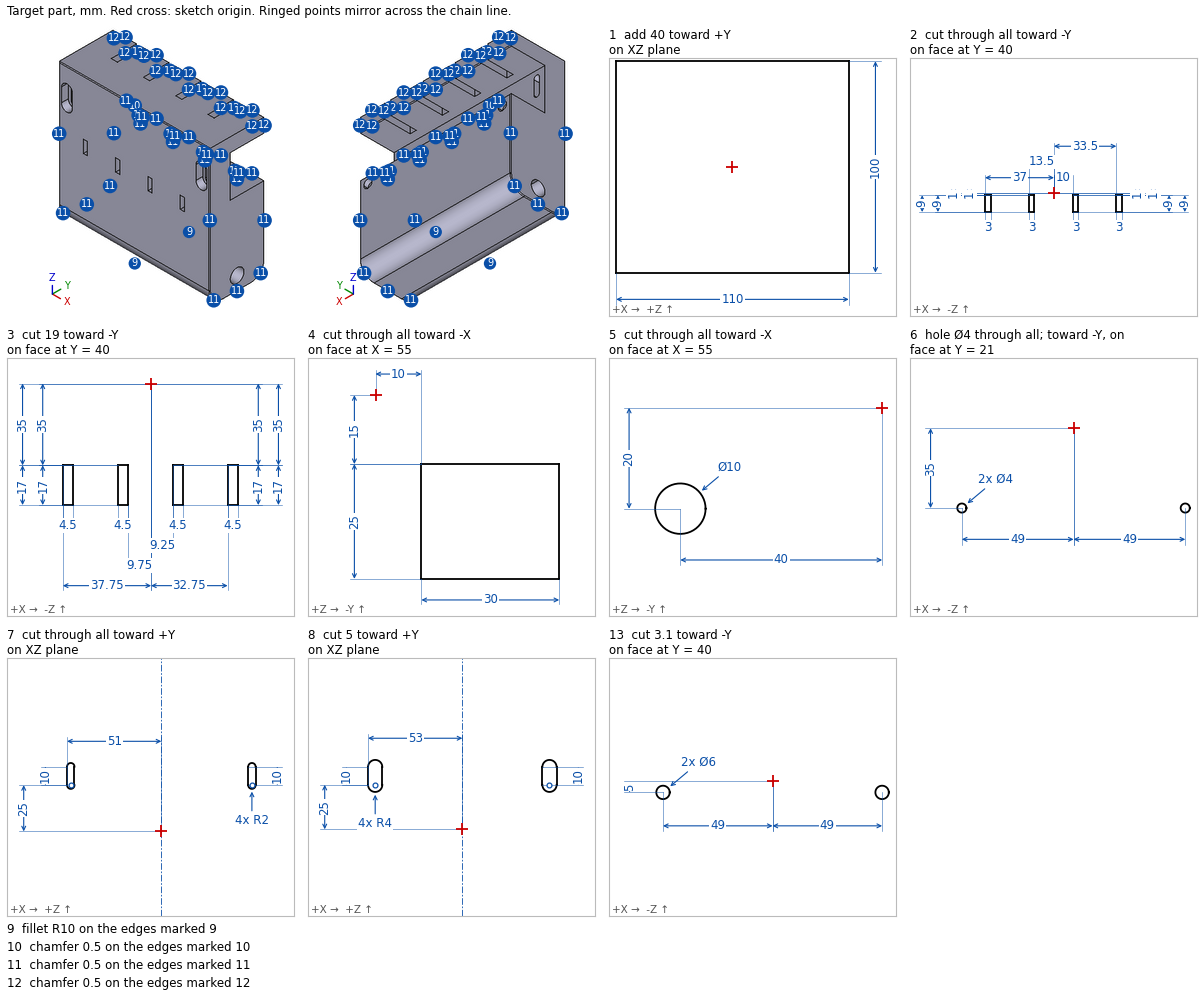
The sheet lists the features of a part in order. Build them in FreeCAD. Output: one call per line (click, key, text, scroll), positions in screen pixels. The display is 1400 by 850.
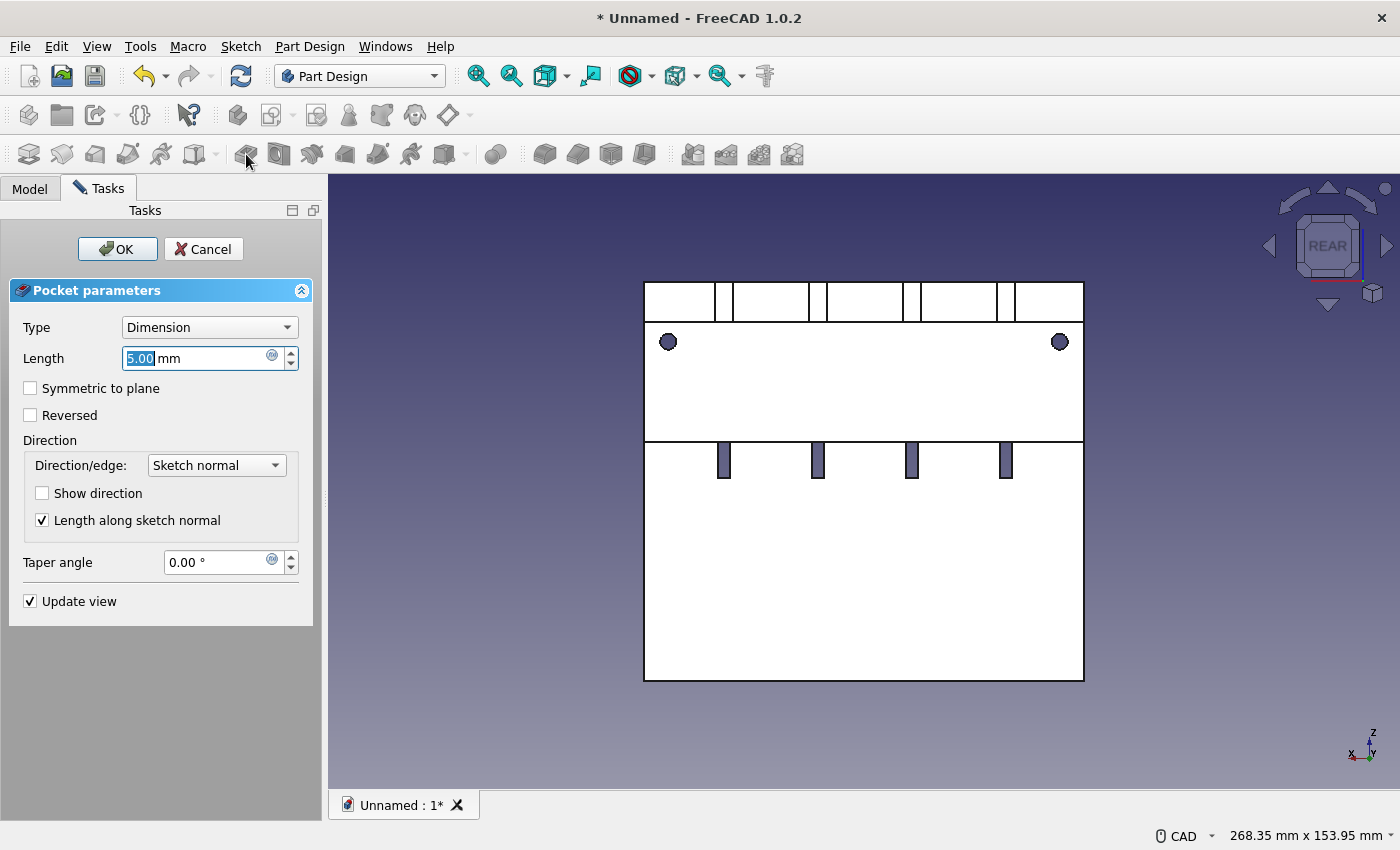
click(210, 328)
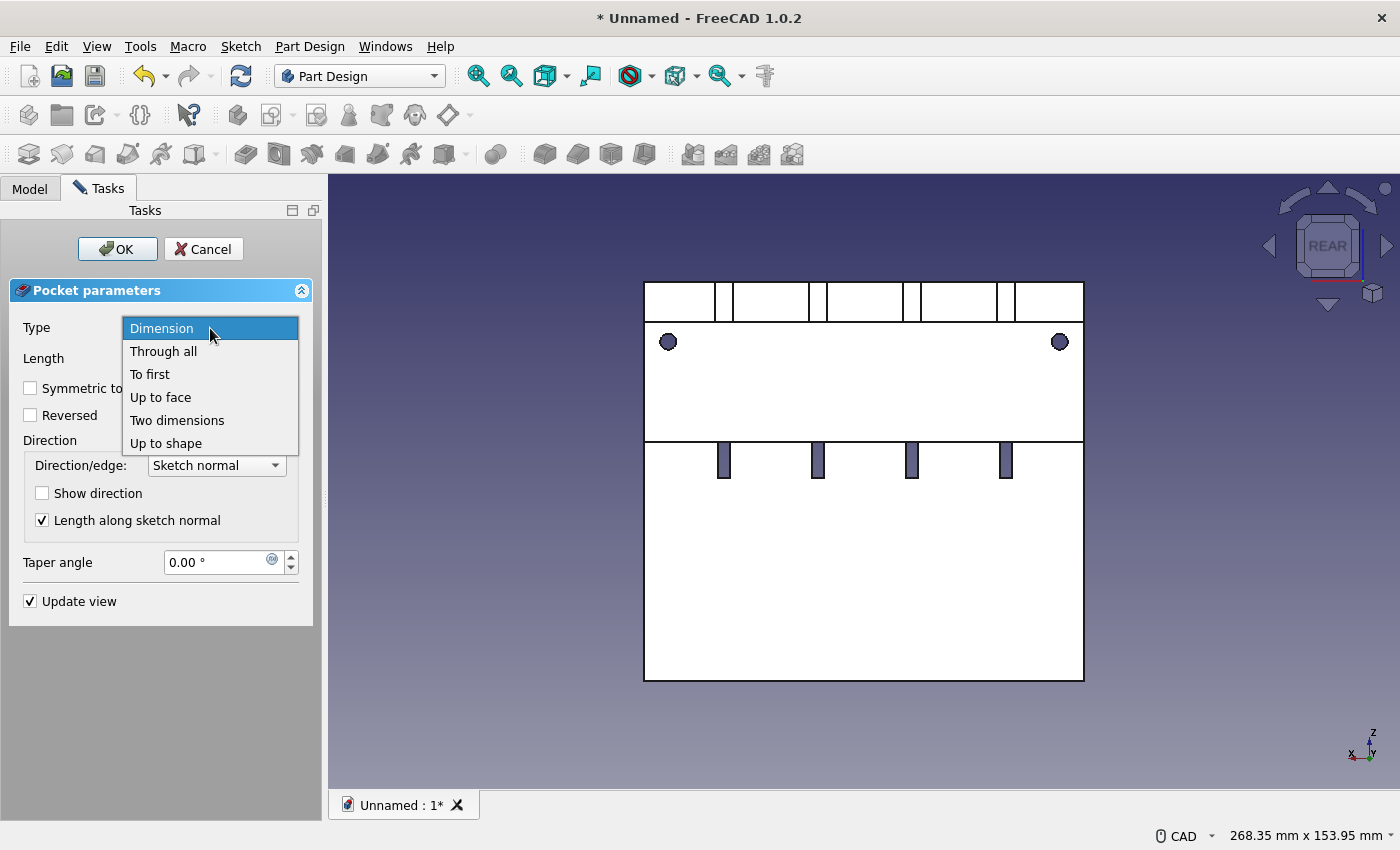
click(208, 352)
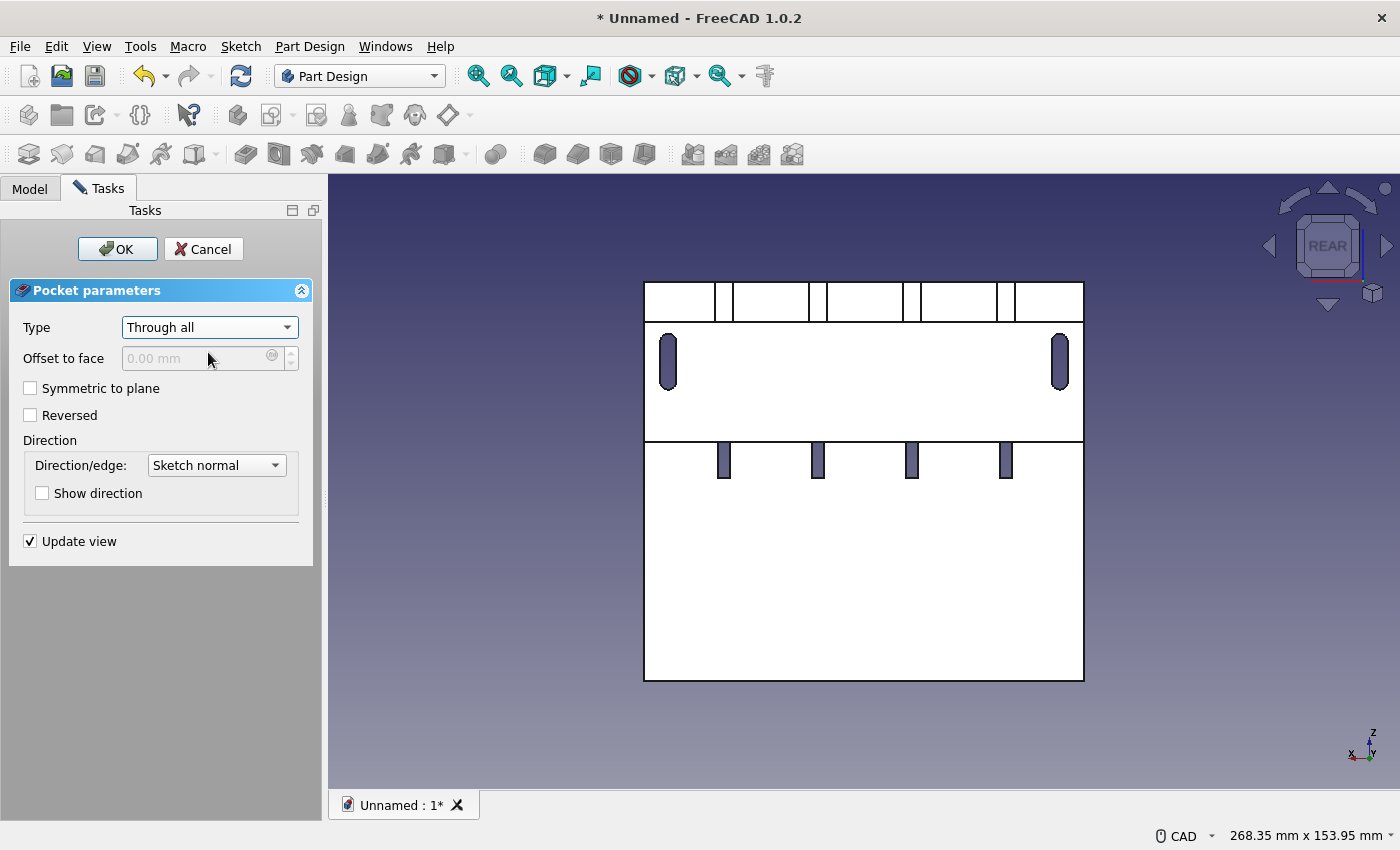
click(118, 249)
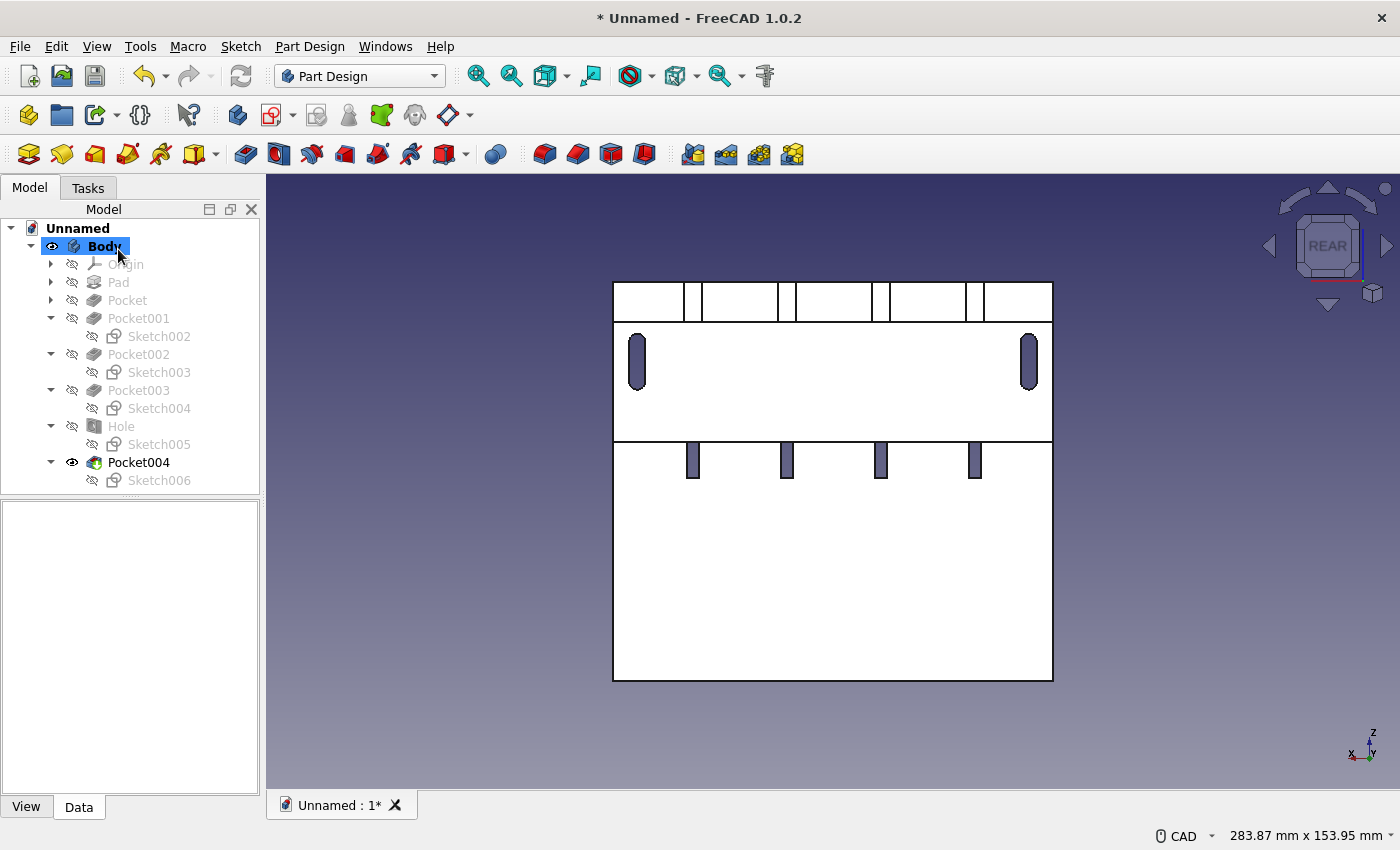
click(270, 116)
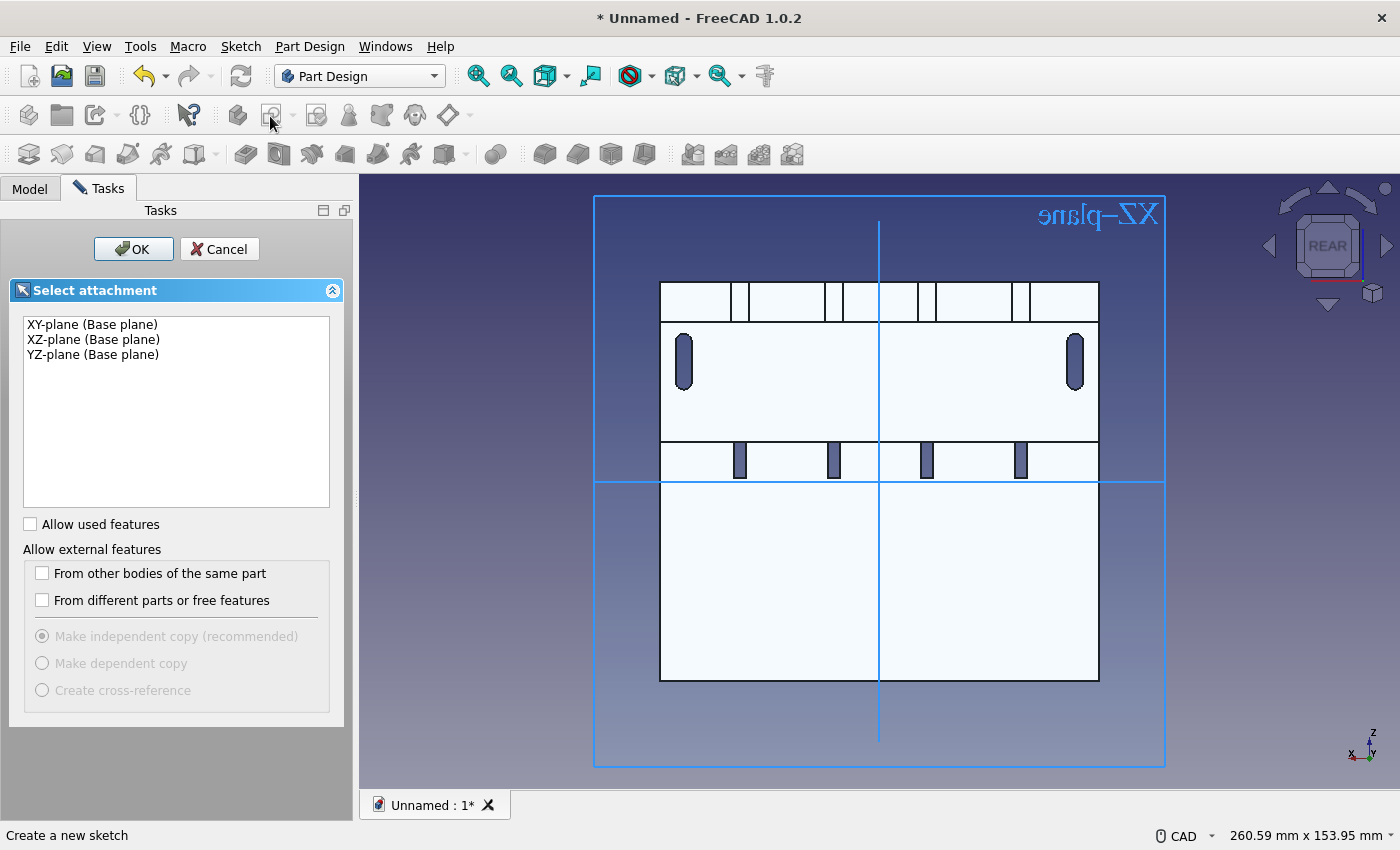
click(84, 340)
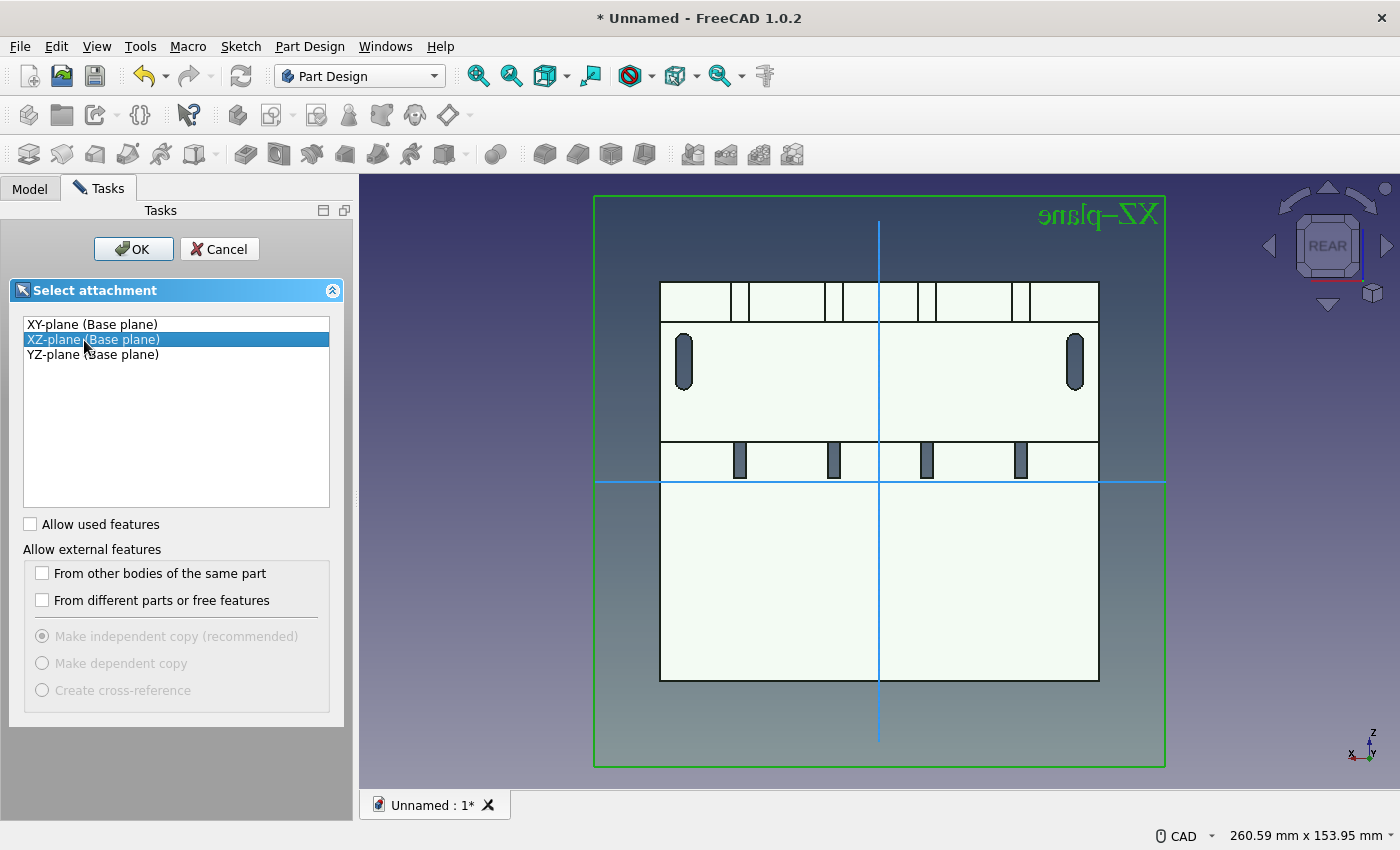
click(134, 249)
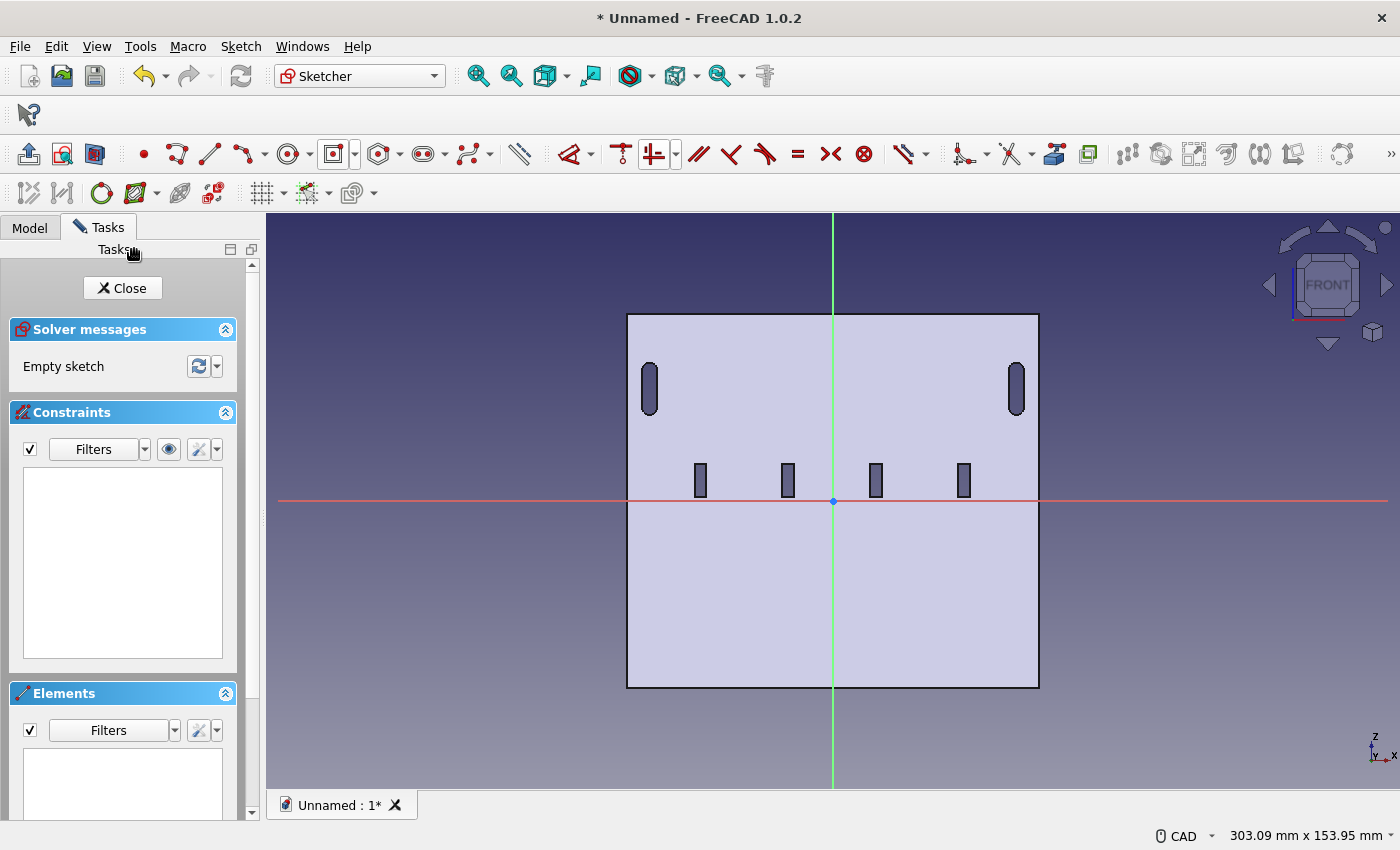
scroll(916, 339, up, 3)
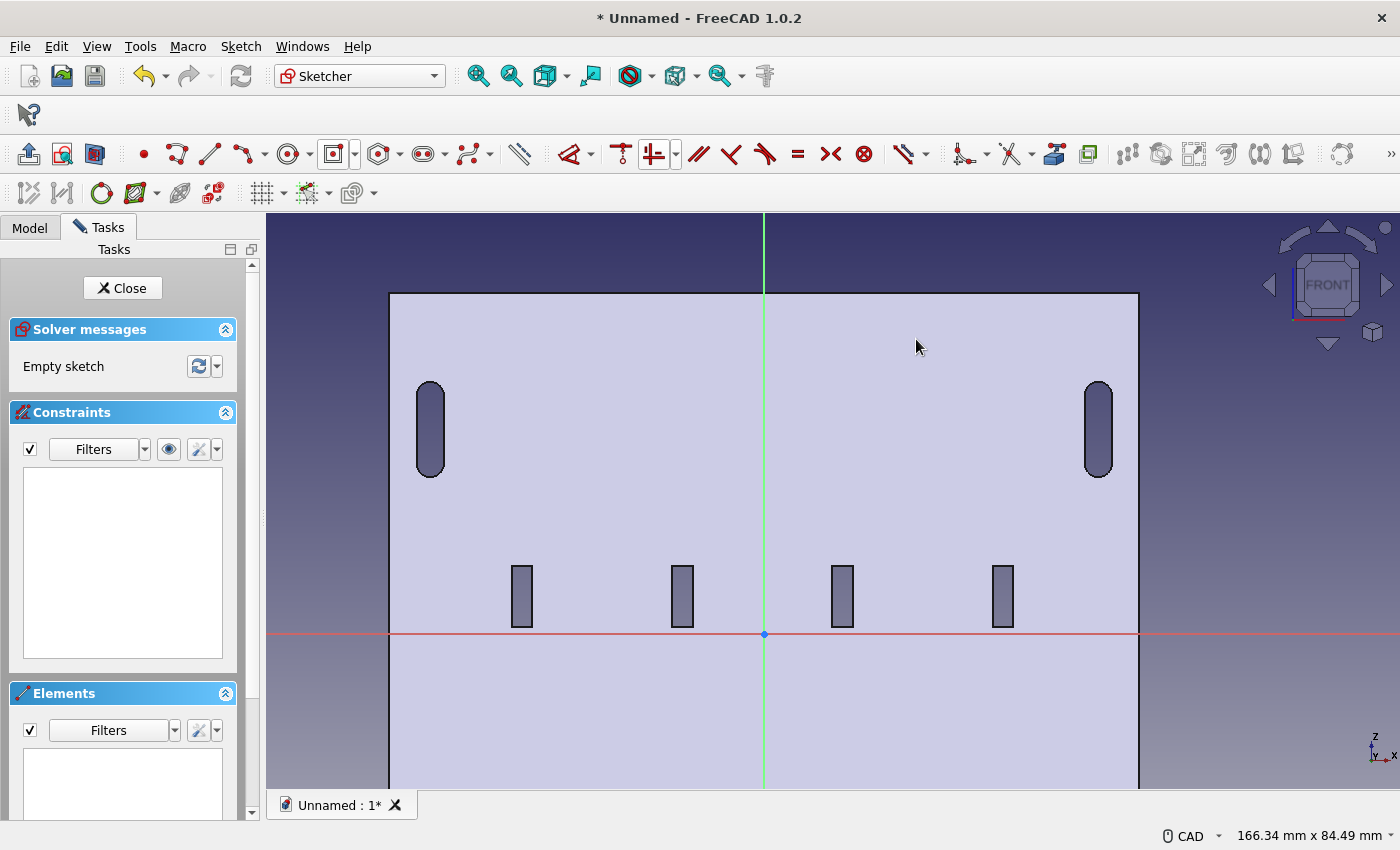
key(g)
key(s)